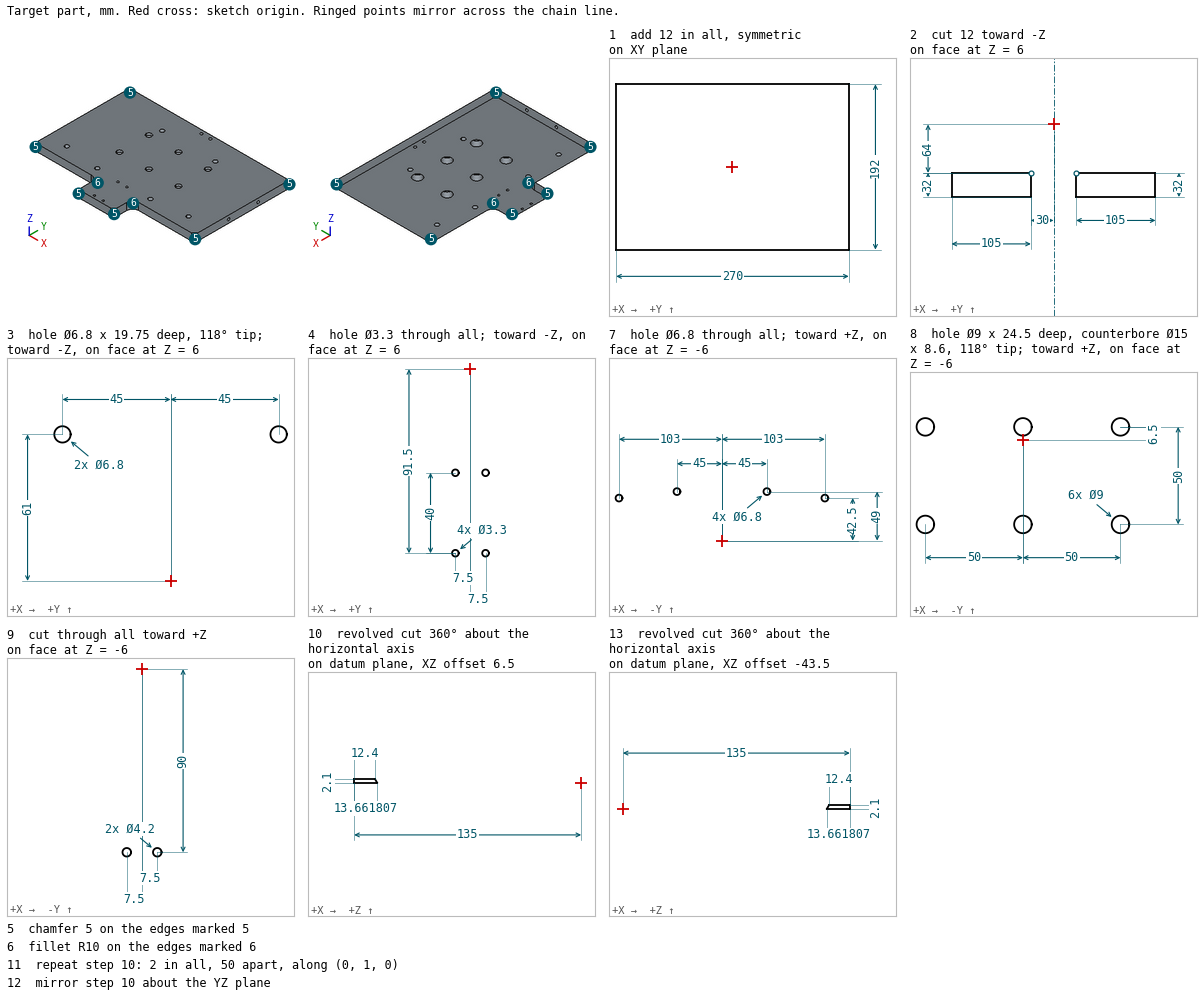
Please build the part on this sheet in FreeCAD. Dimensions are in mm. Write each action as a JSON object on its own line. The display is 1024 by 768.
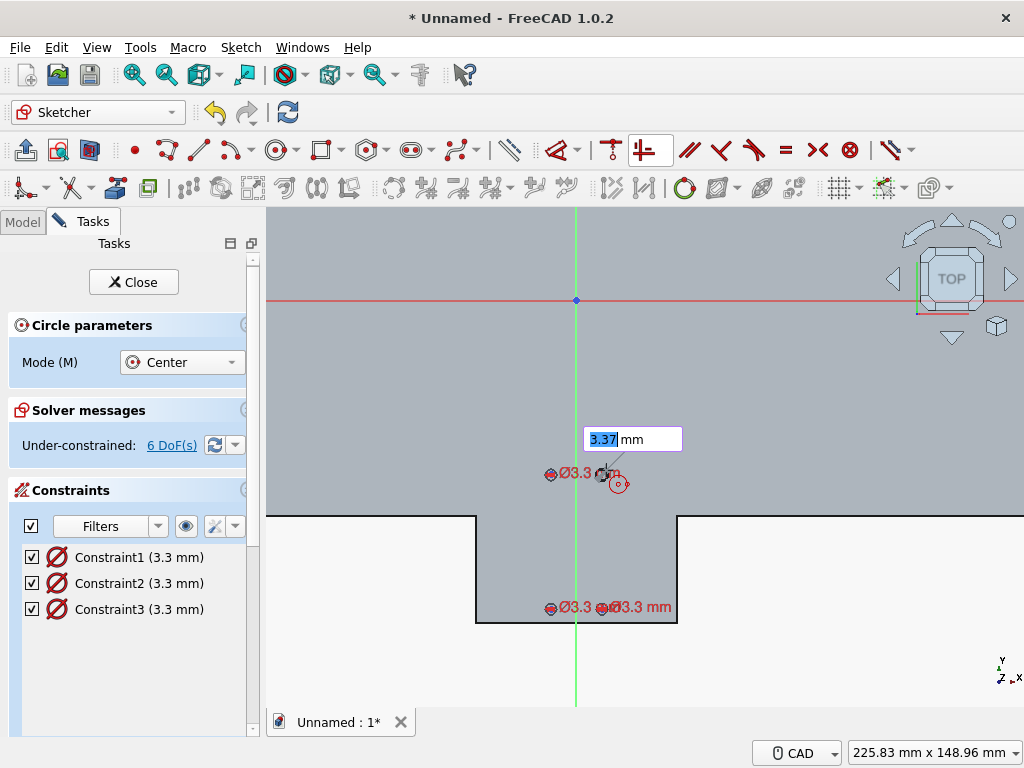
{"action": "type", "text": "3.3"}
{"action": "key", "text": "Return"}
{"action": "key", "text": "Escape"}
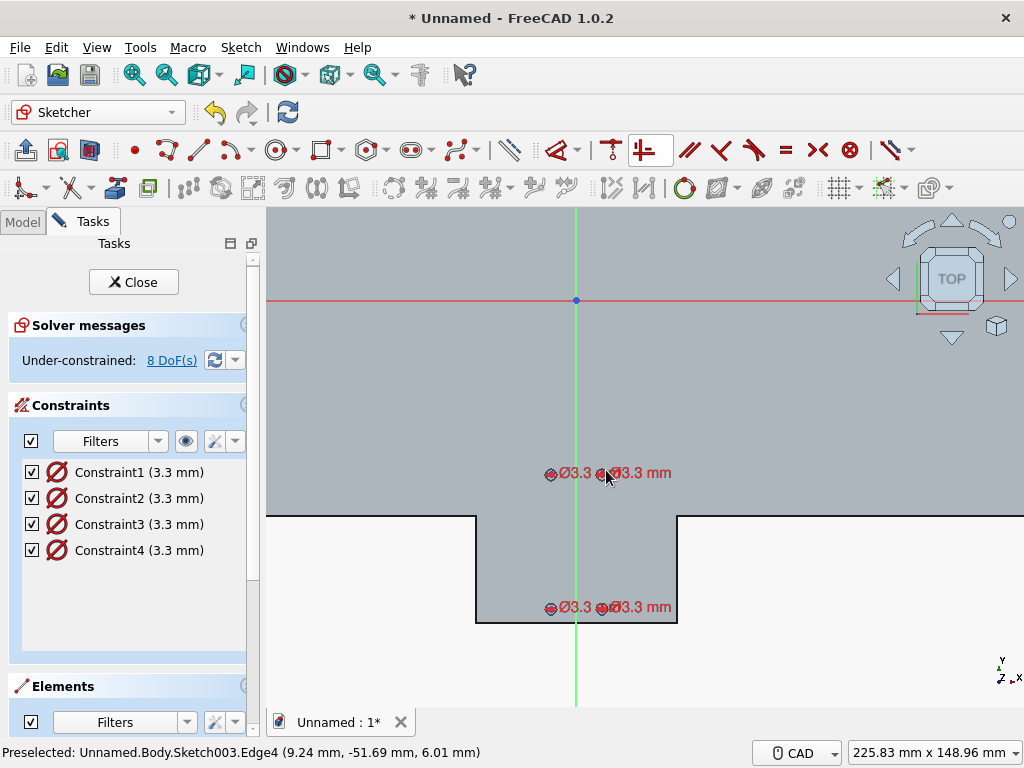
{"action": "left_click", "coordinate": [551, 609]}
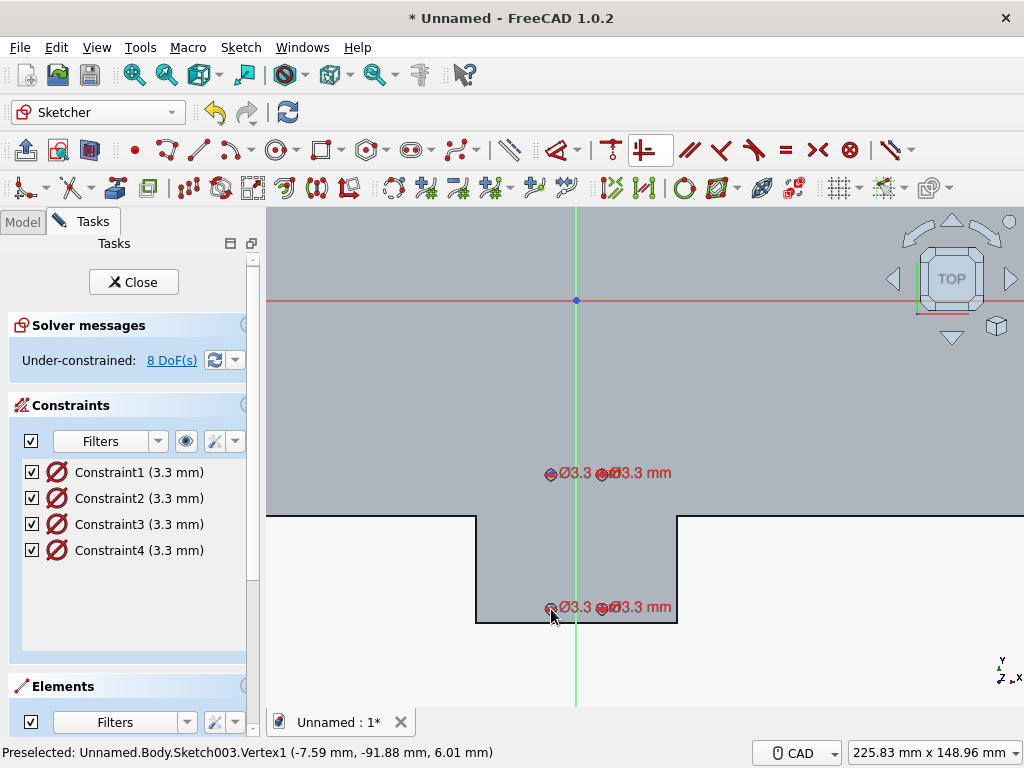
{"action": "left_click", "coordinate": [602, 609]}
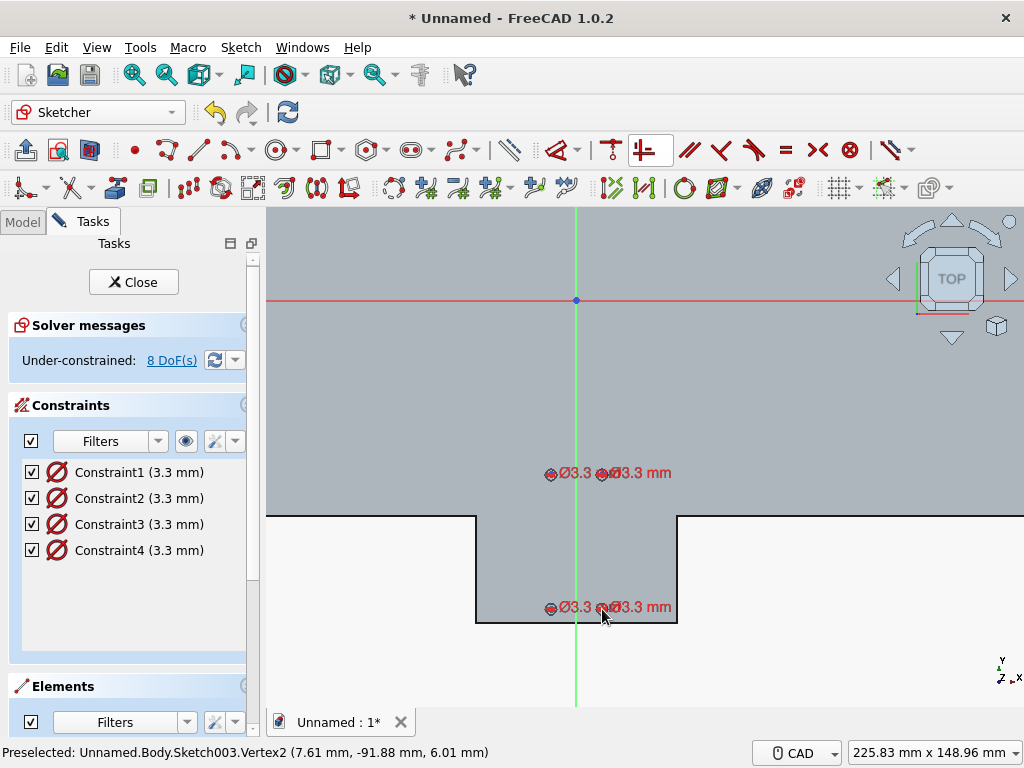
{"action": "key", "text": "h"}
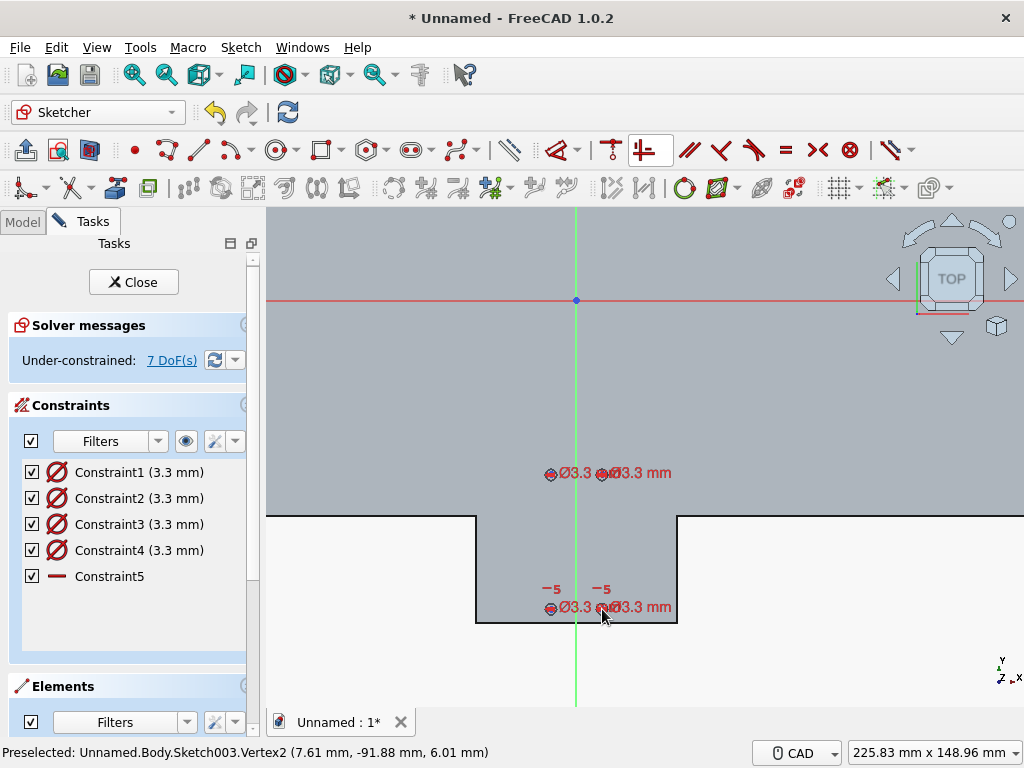
{"action": "left_click", "coordinate": [551, 609]}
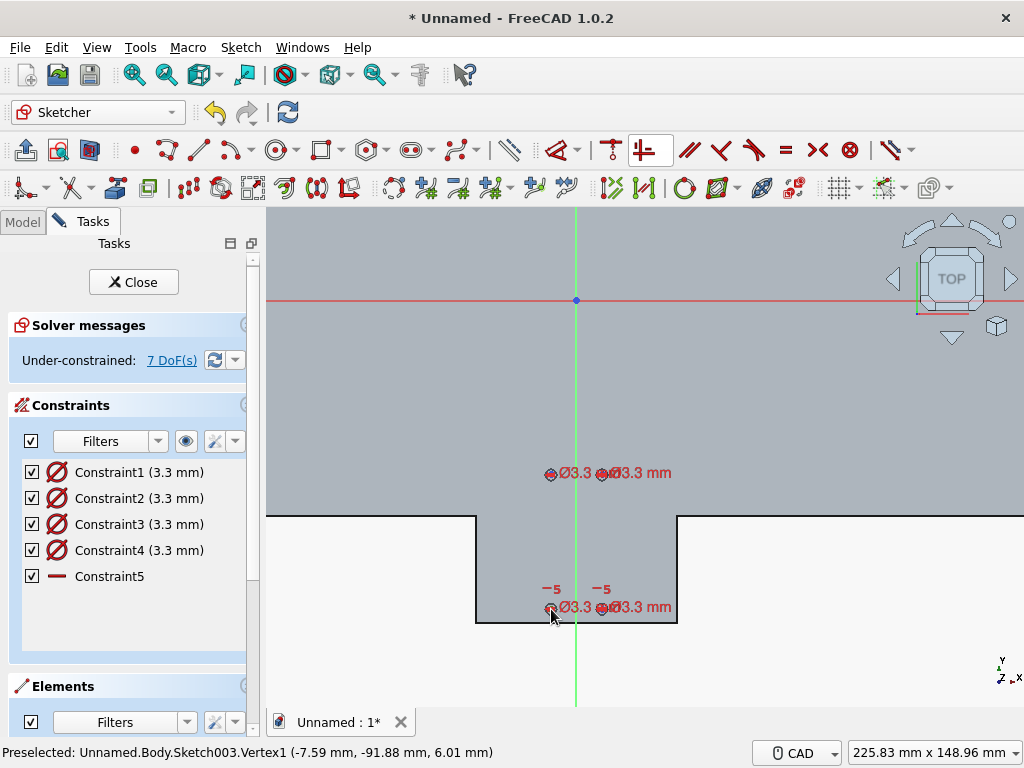
{"action": "left_click", "coordinate": [551, 475]}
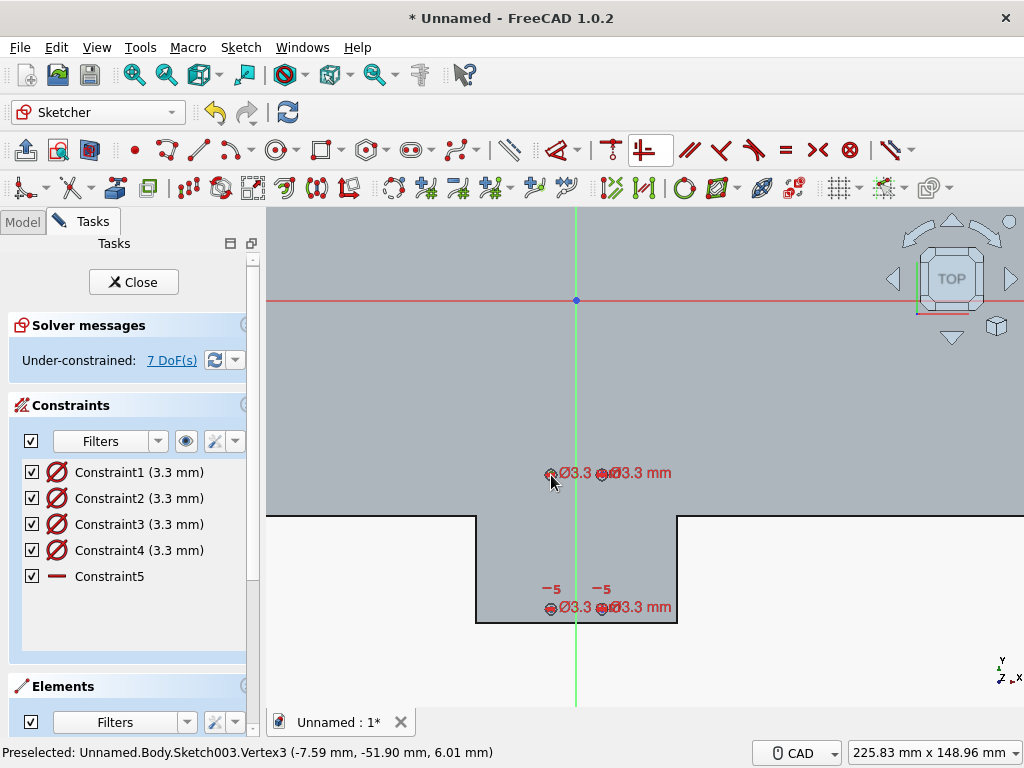
{"action": "key", "text": "v"}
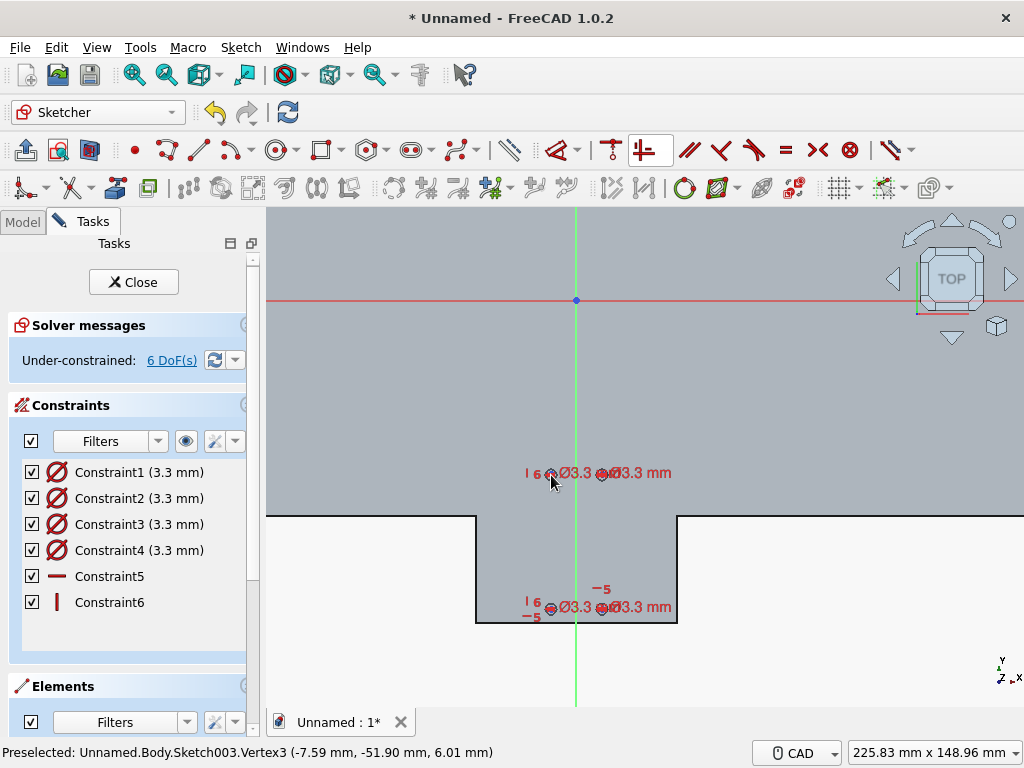
{"action": "left_click", "coordinate": [602, 609]}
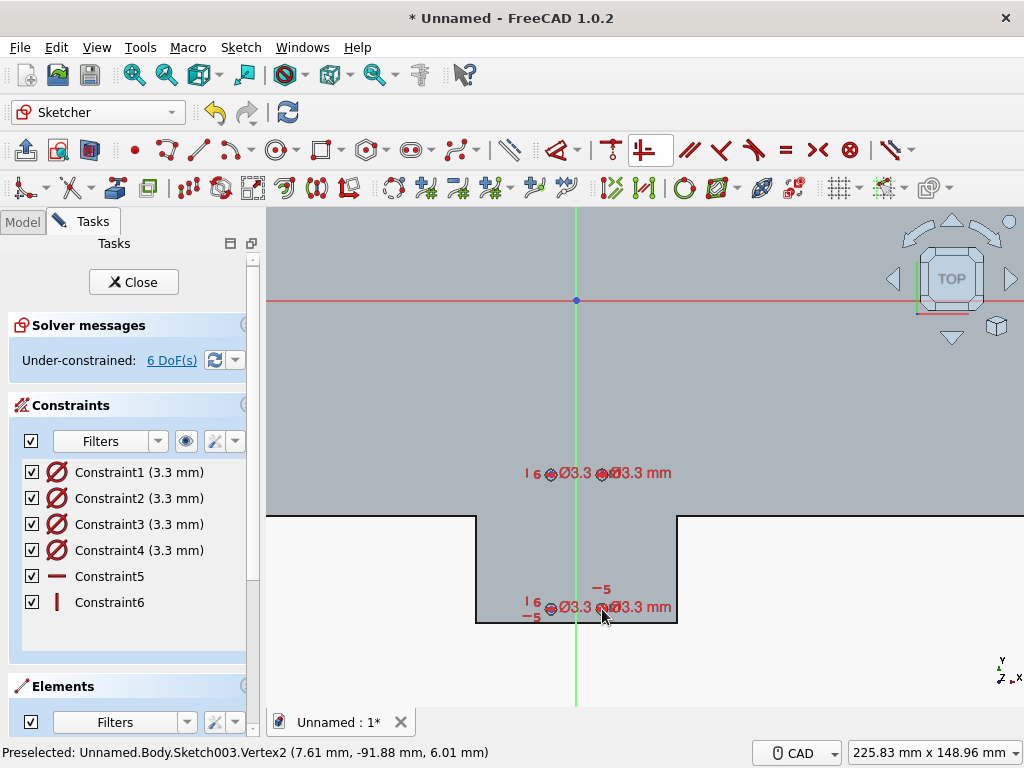
{"action": "left_click", "coordinate": [602, 475]}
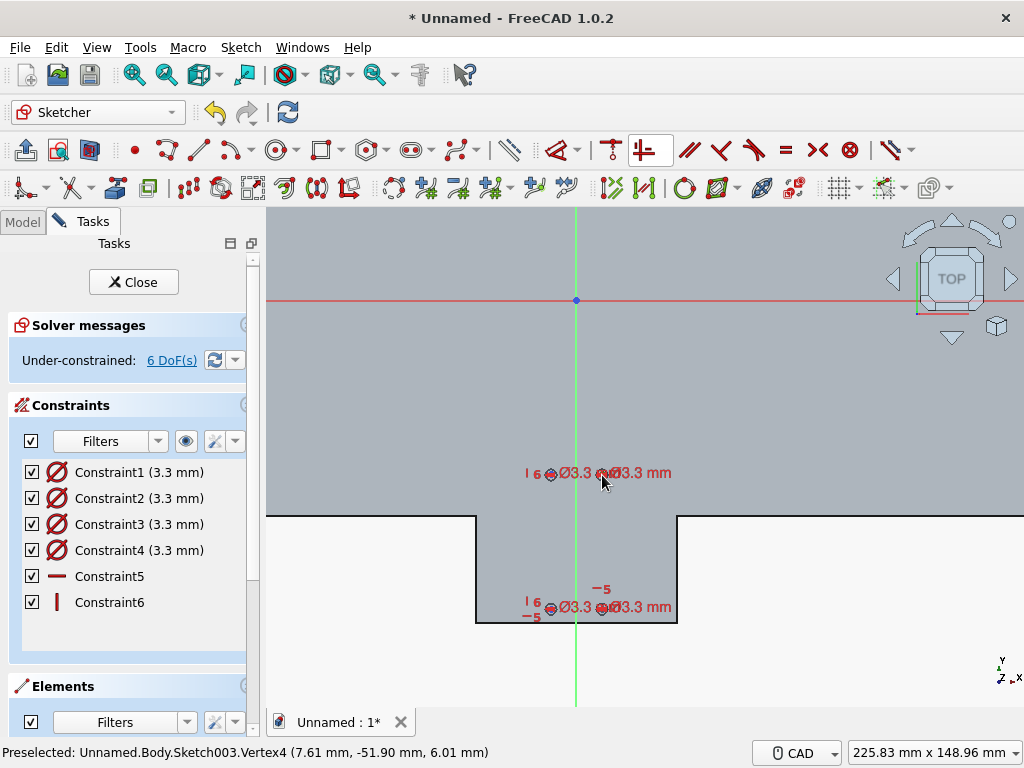
{"action": "key", "text": "v"}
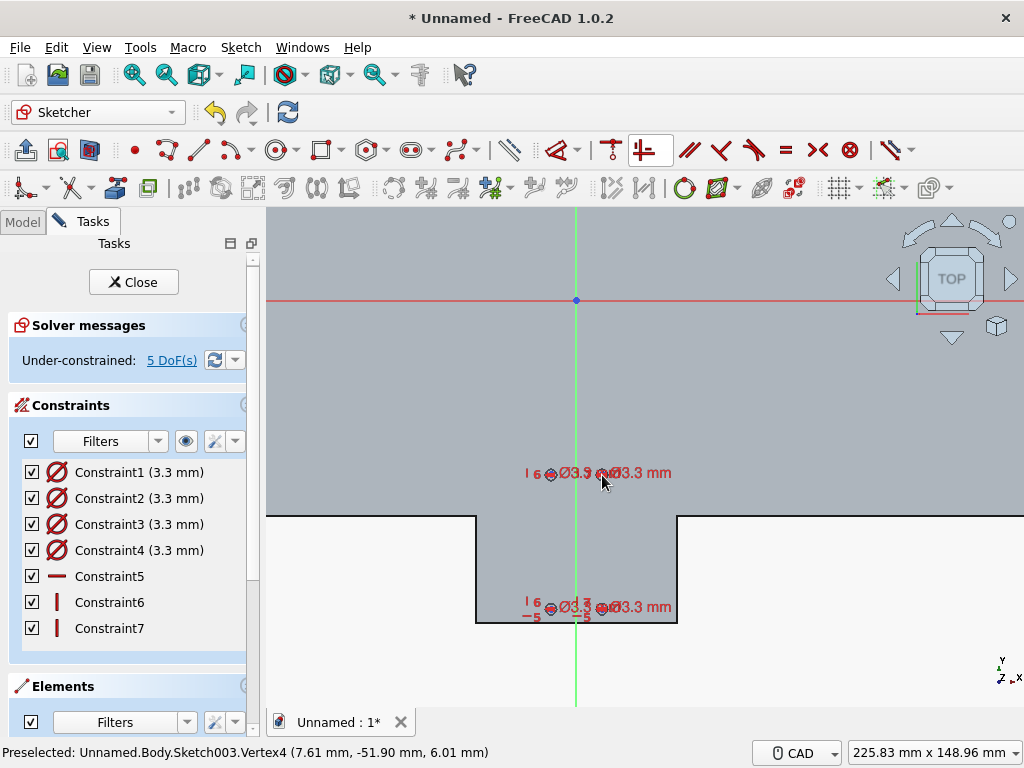
{"action": "left_click", "coordinate": [551, 475]}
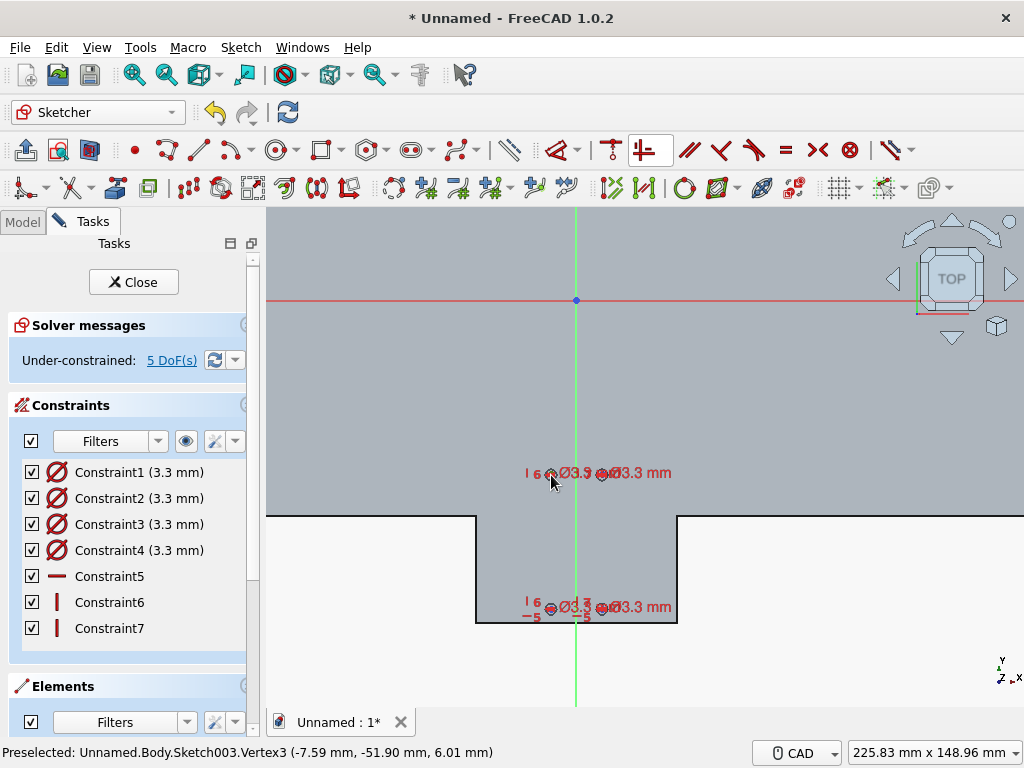
{"action": "left_click", "coordinate": [602, 475]}